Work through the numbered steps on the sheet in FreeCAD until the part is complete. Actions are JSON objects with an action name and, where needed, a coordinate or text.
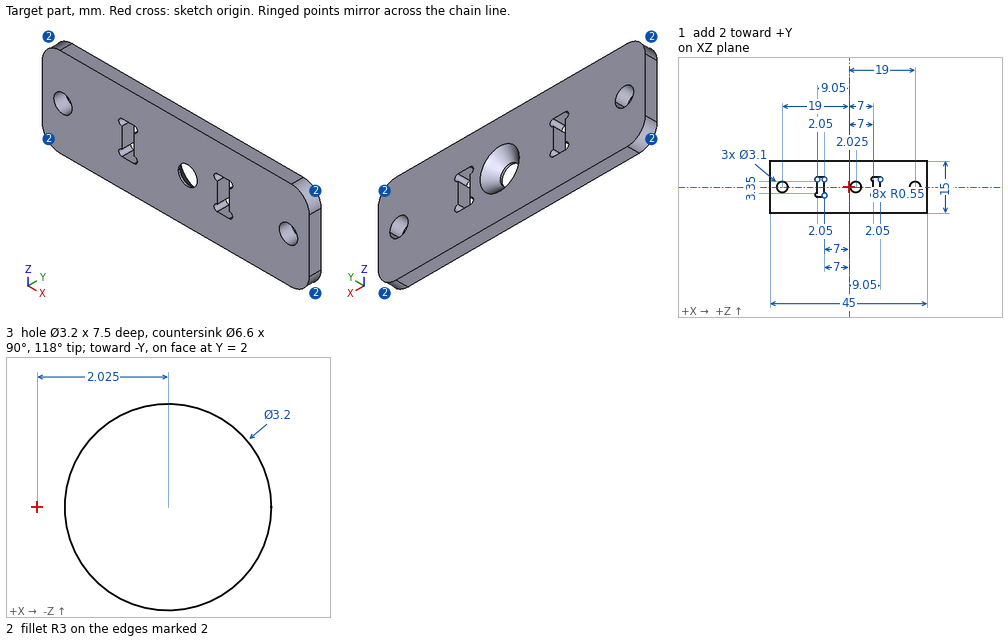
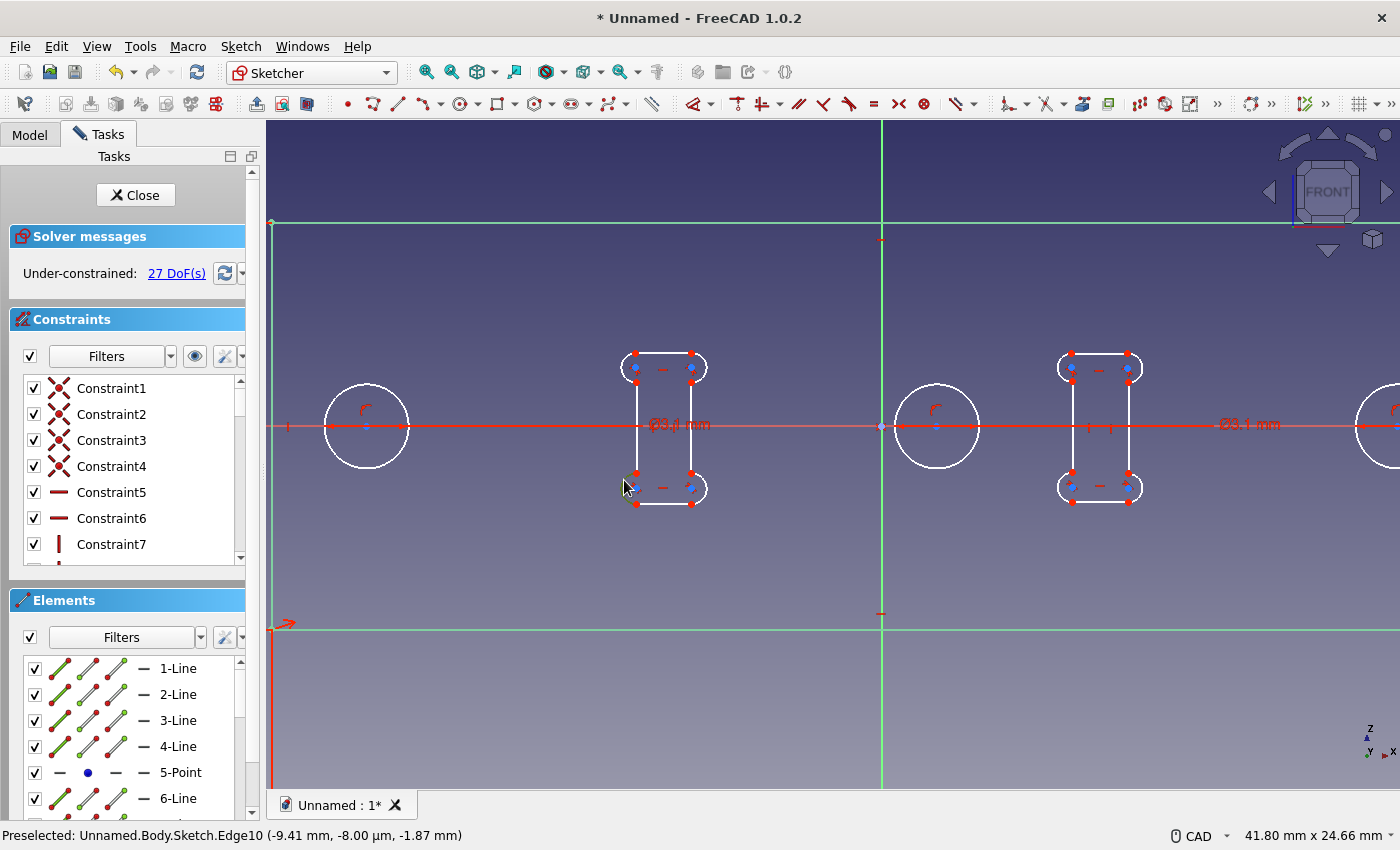
{"action": "left_click", "coordinate": [704, 498]}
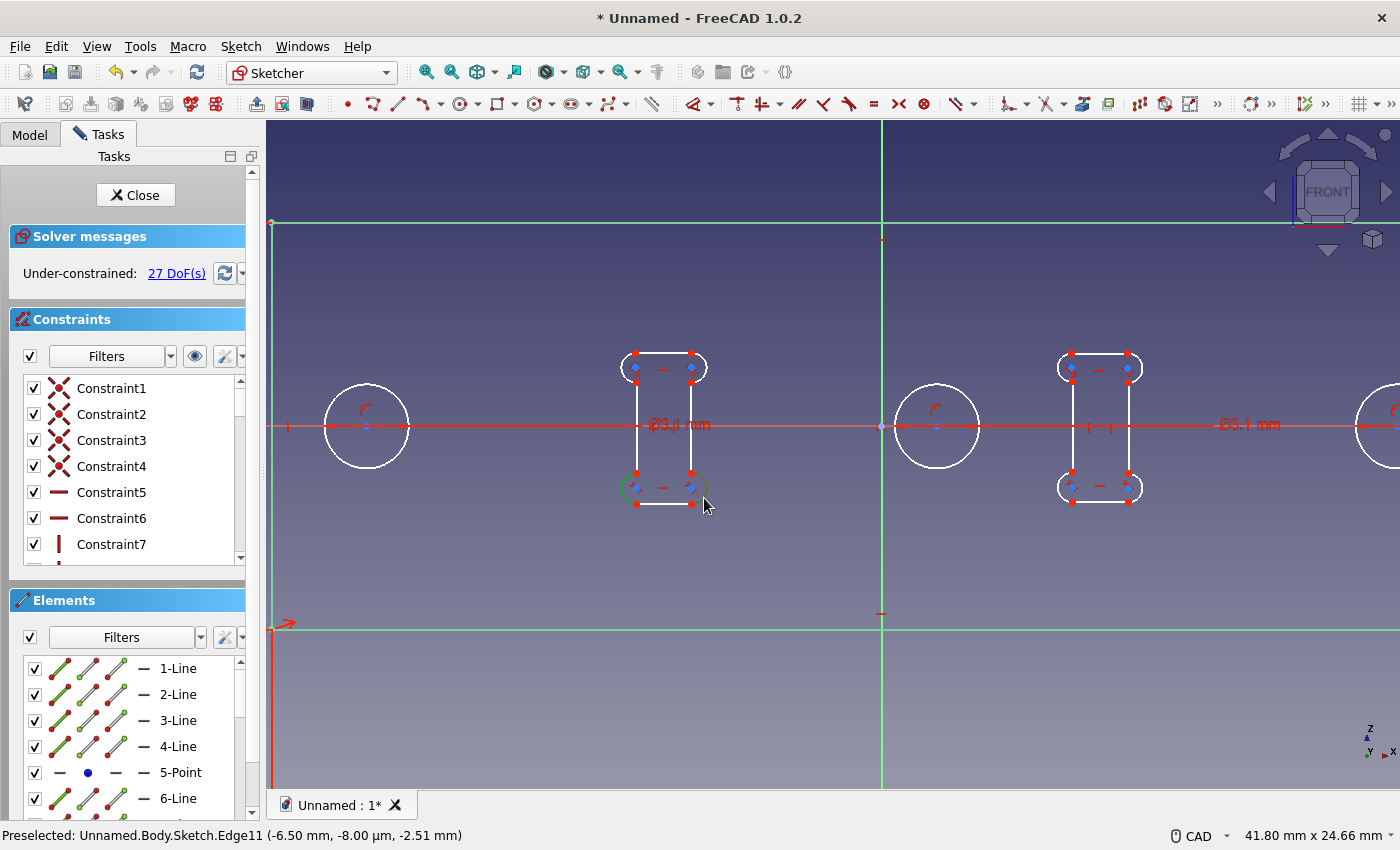
{"action": "left_click", "coordinate": [703, 377]}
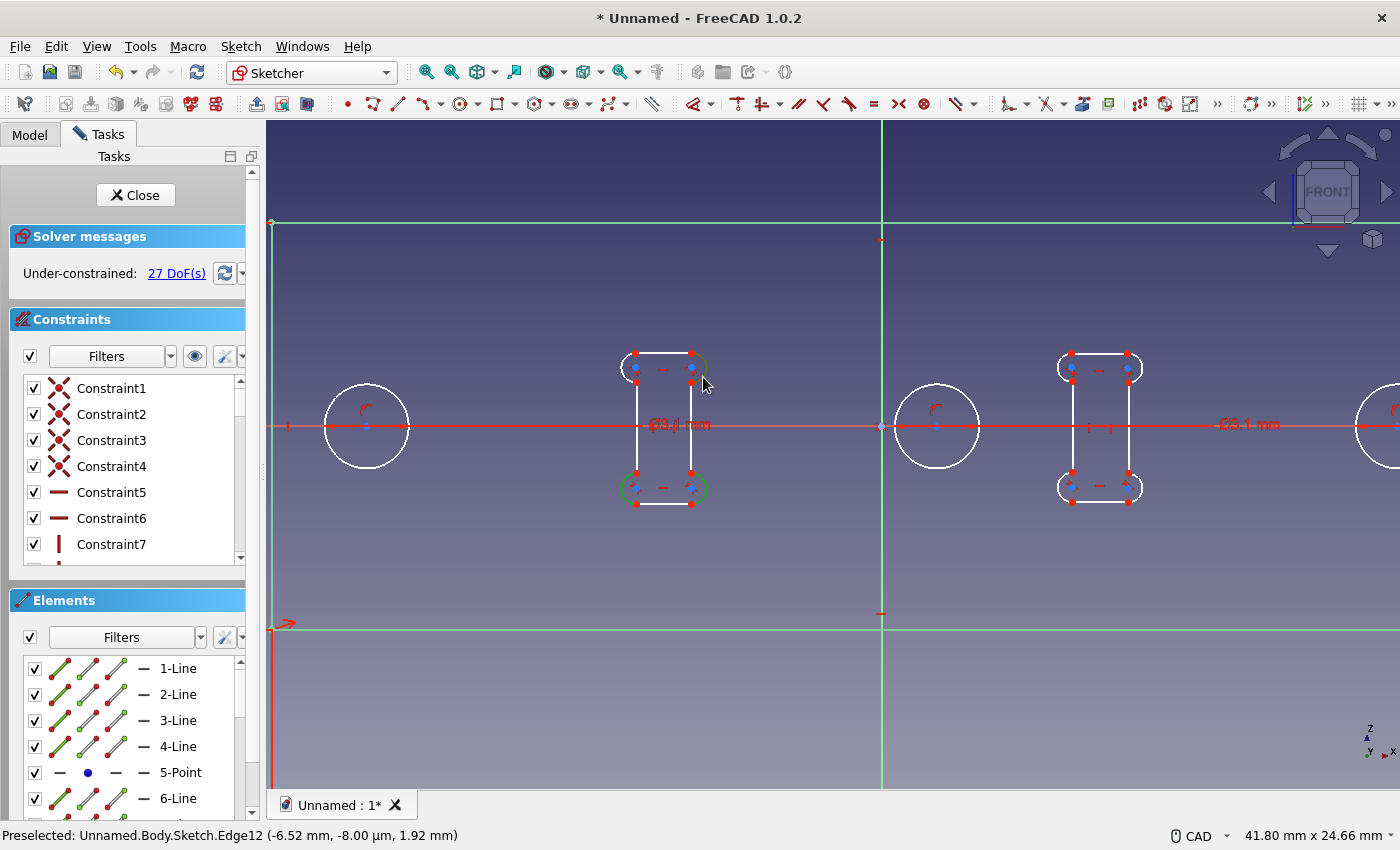
{"action": "left_click", "coordinate": [624, 359]}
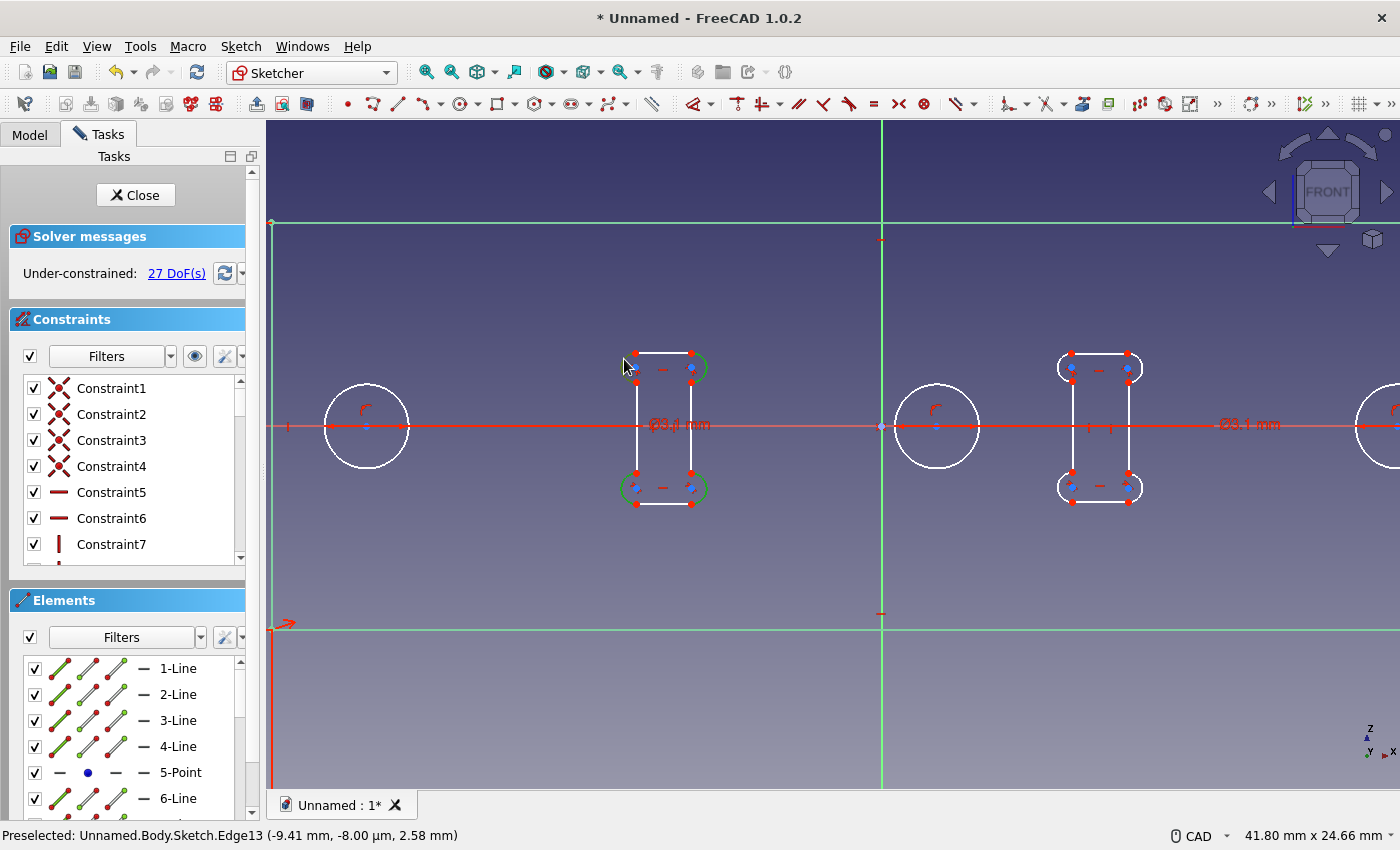
{"action": "left_click", "coordinate": [1061, 479]}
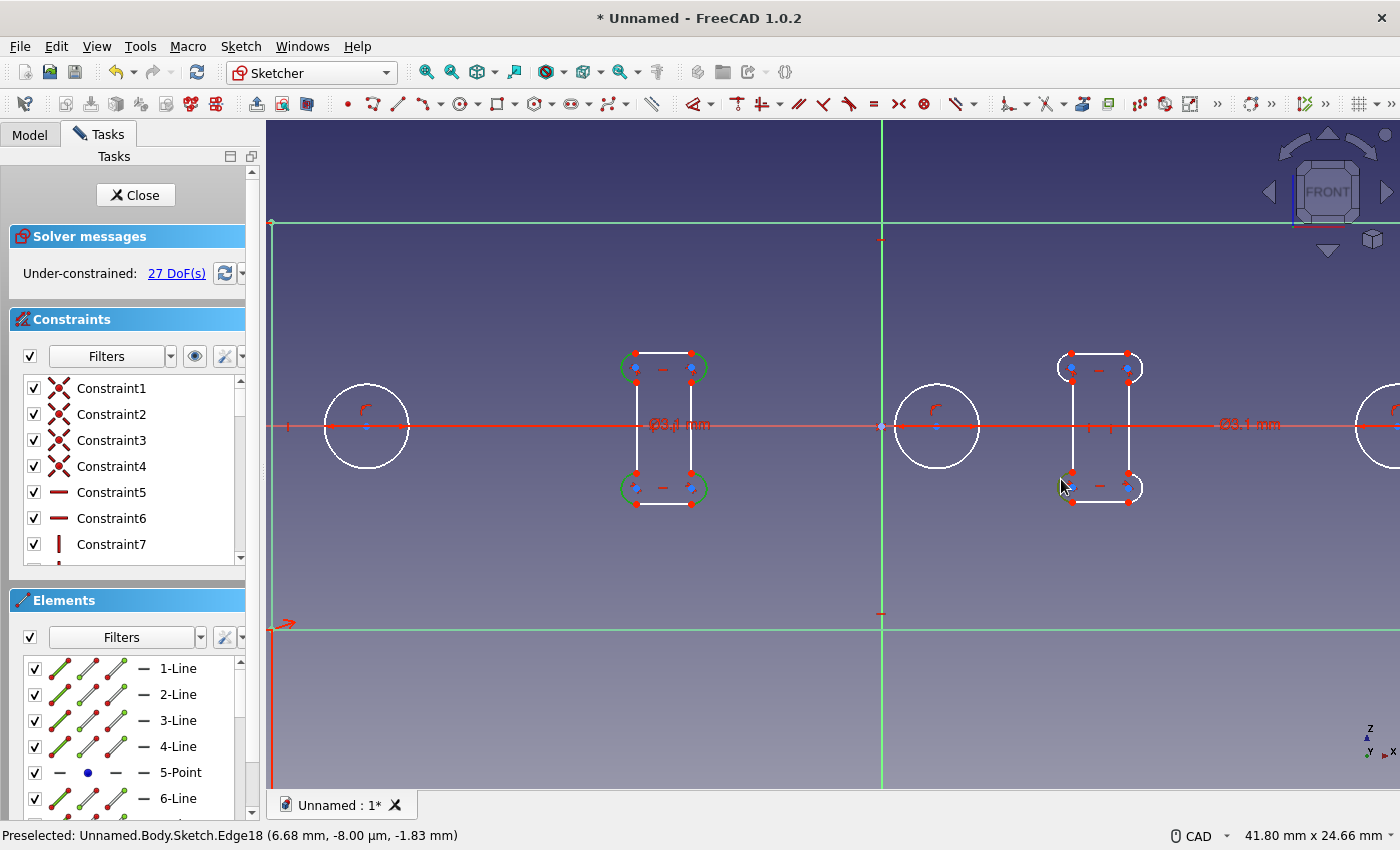
{"action": "left_click", "coordinate": [1140, 496]}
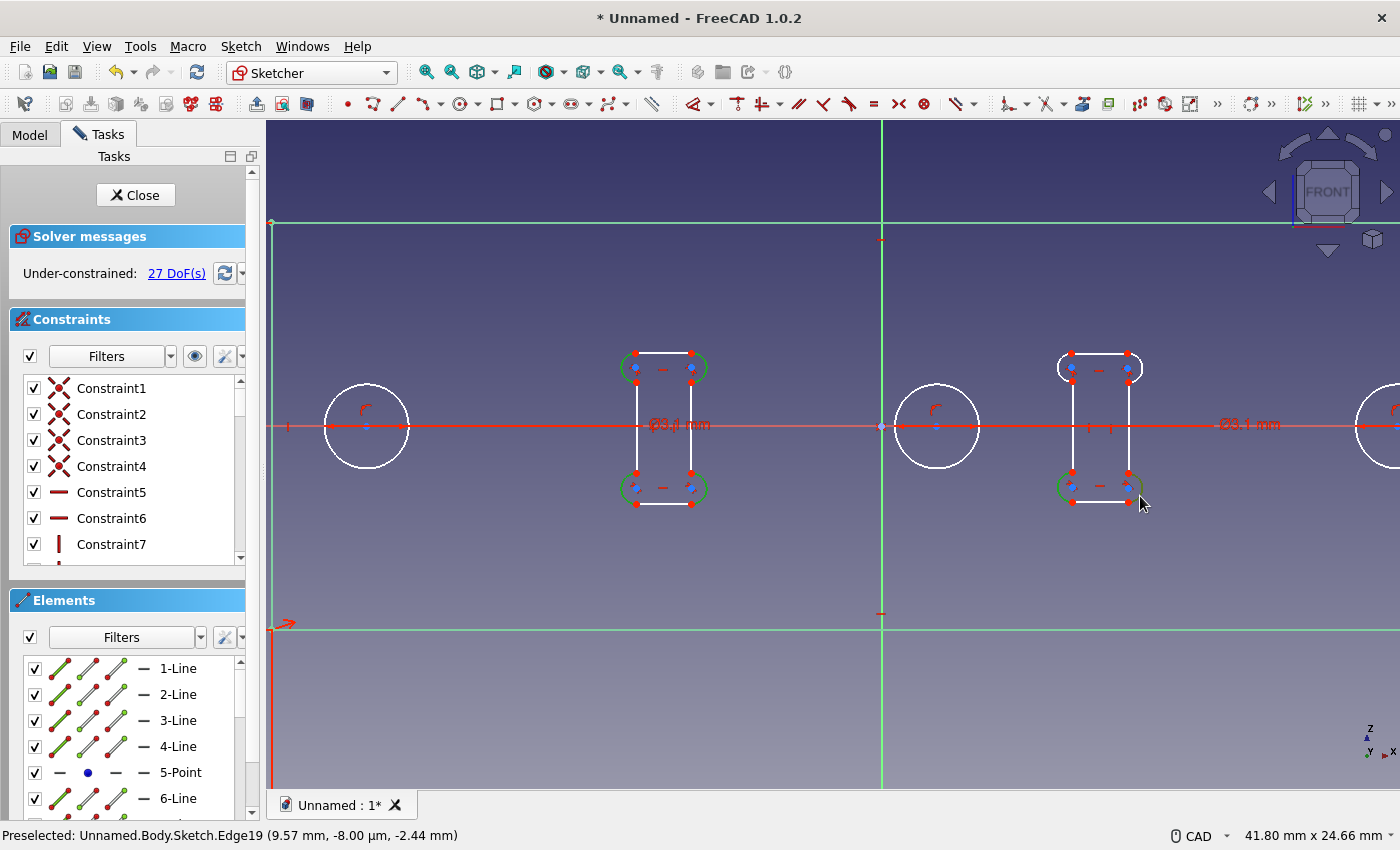
{"action": "left_click", "coordinate": [1140, 376]}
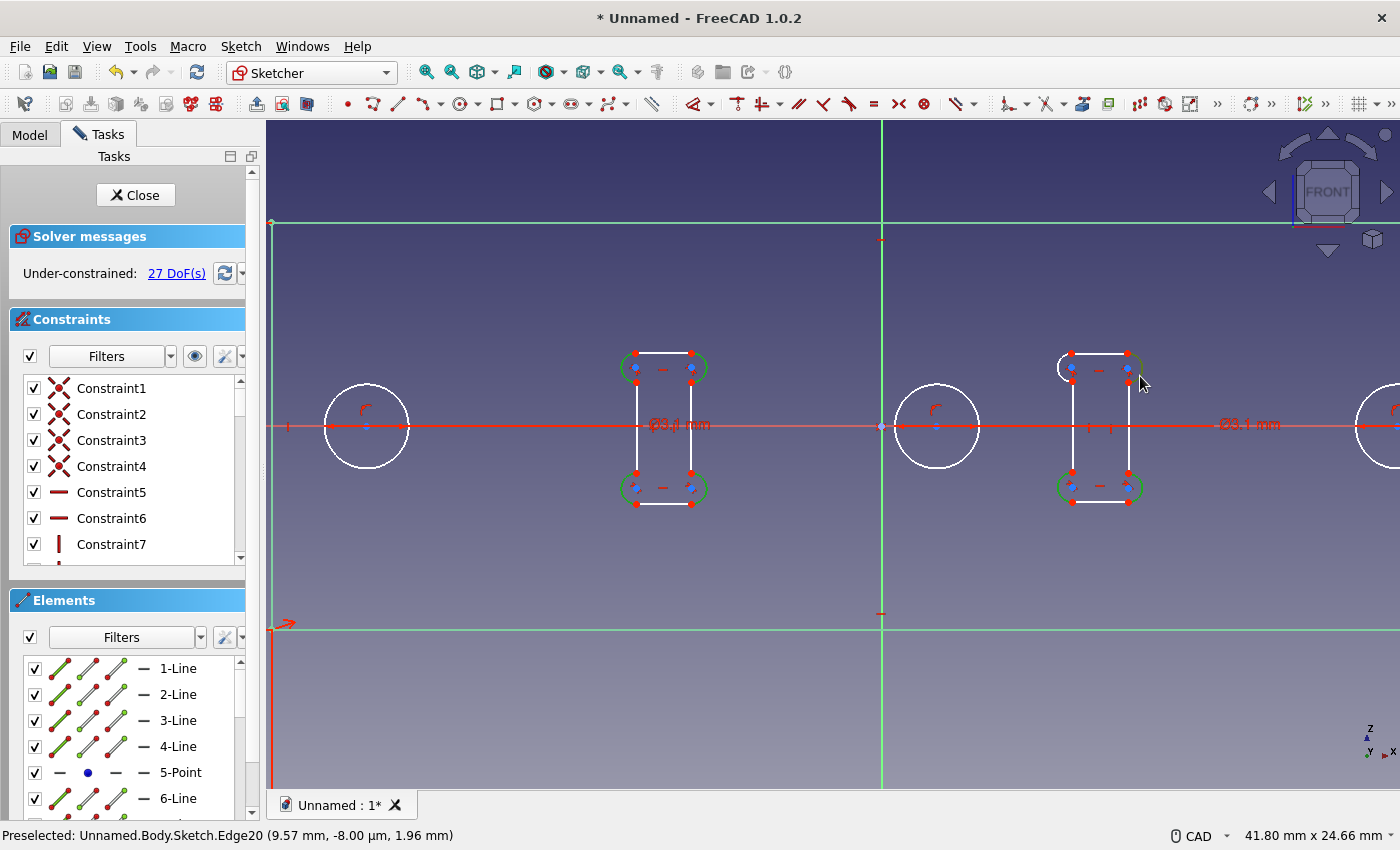
{"action": "left_click", "coordinate": [1060, 360]}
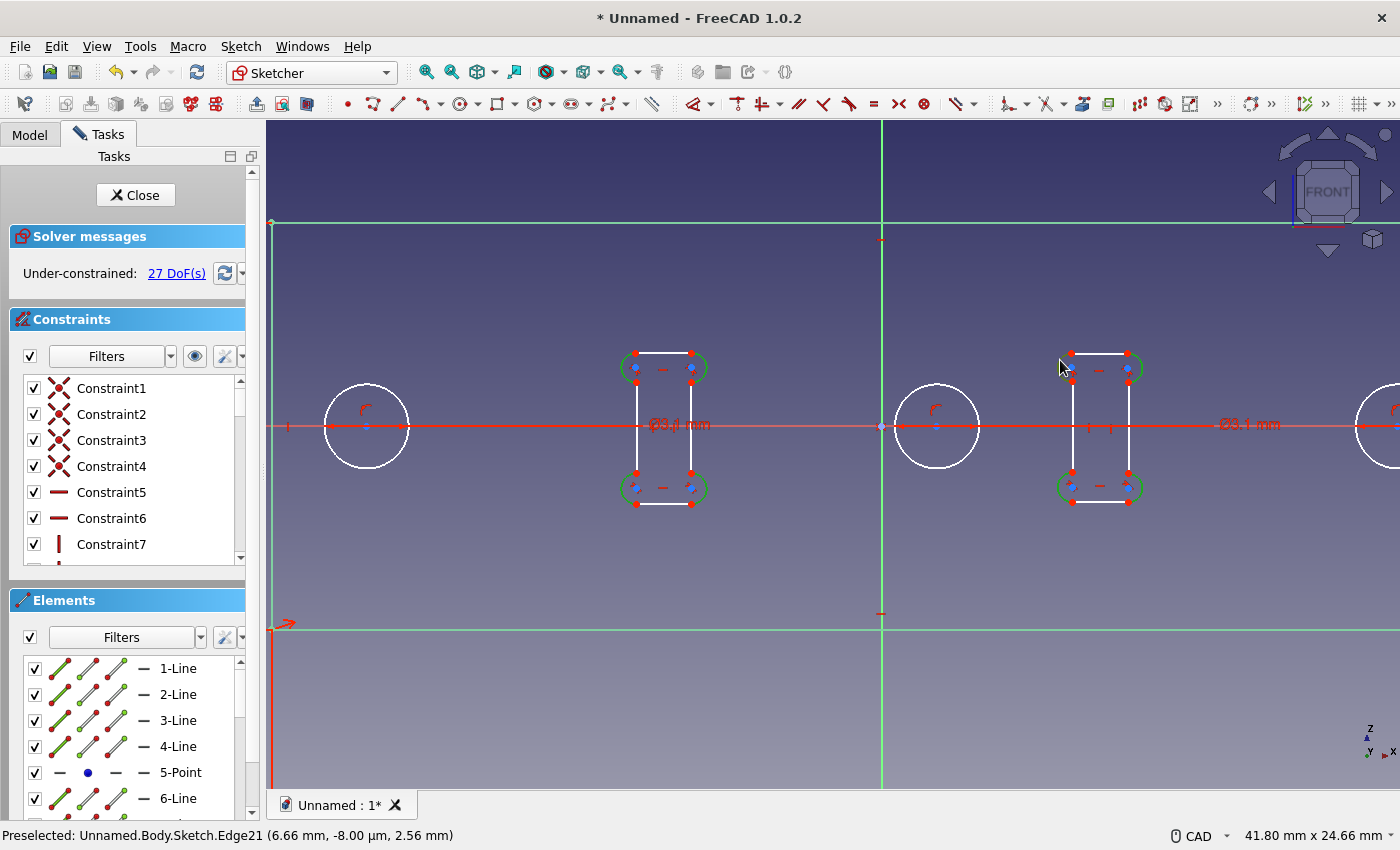
{"action": "left_click", "coordinate": [874, 104]}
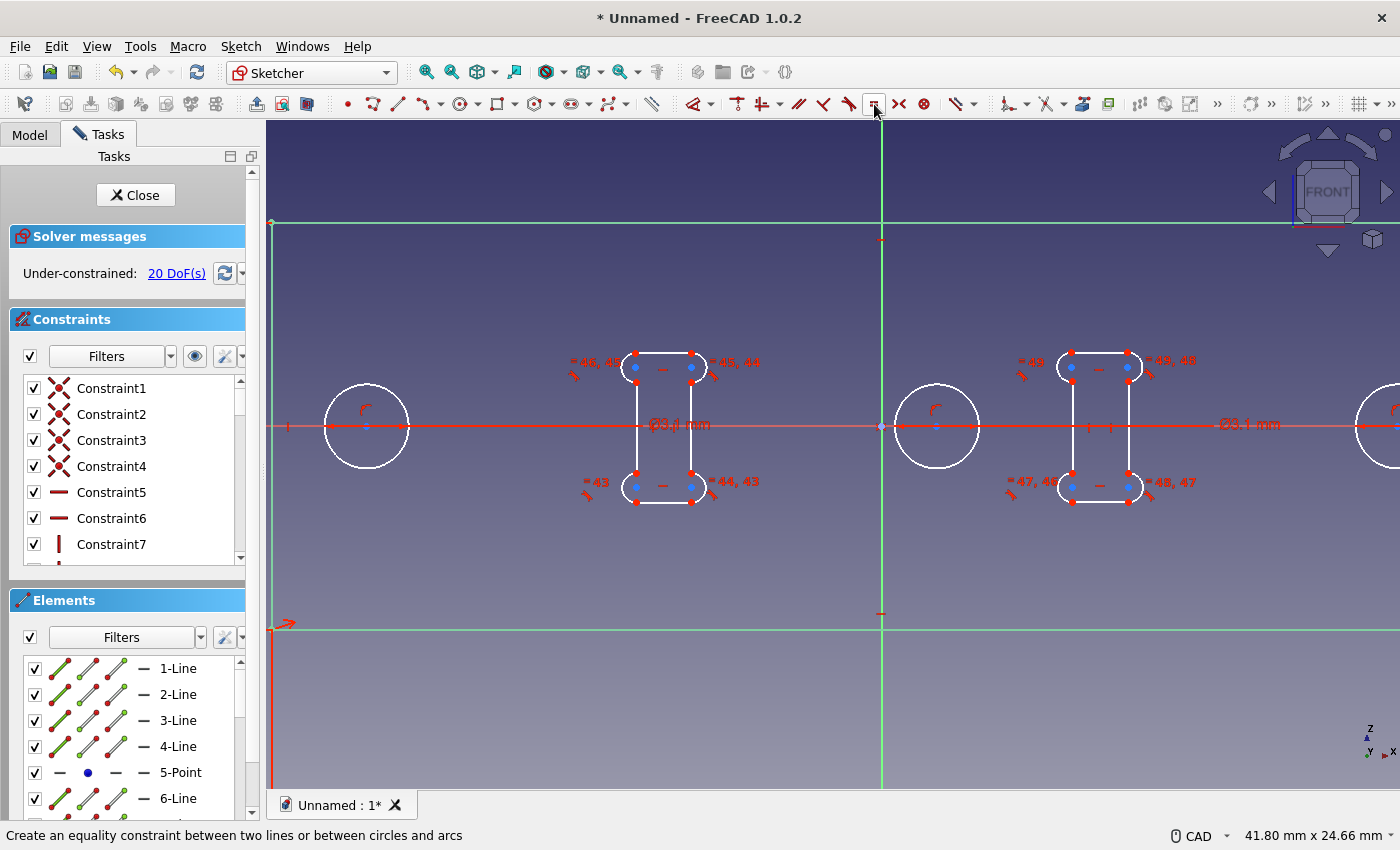
{"action": "left_click", "coordinate": [691, 488]}